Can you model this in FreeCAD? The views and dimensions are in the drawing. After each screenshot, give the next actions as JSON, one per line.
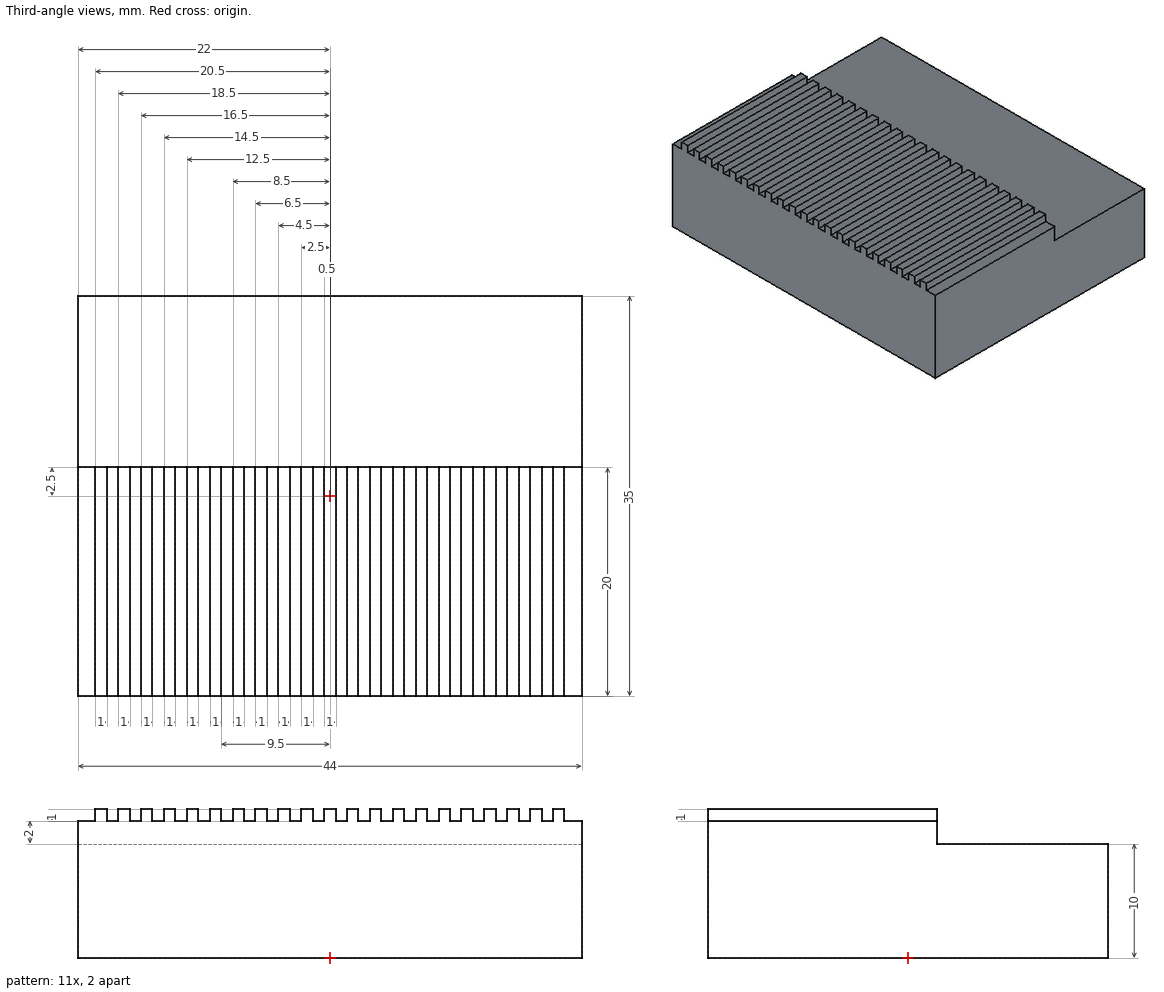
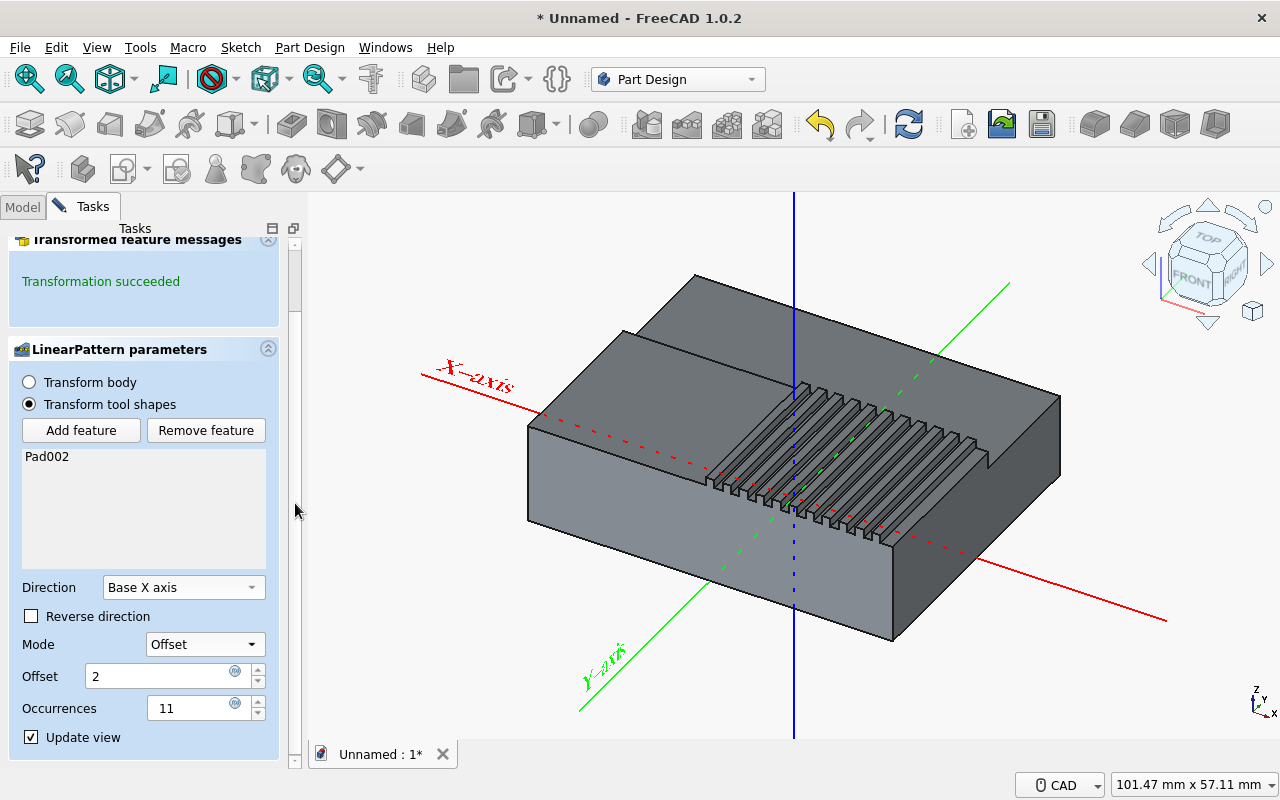
{"action": "left_click", "coordinate": [96, 267]}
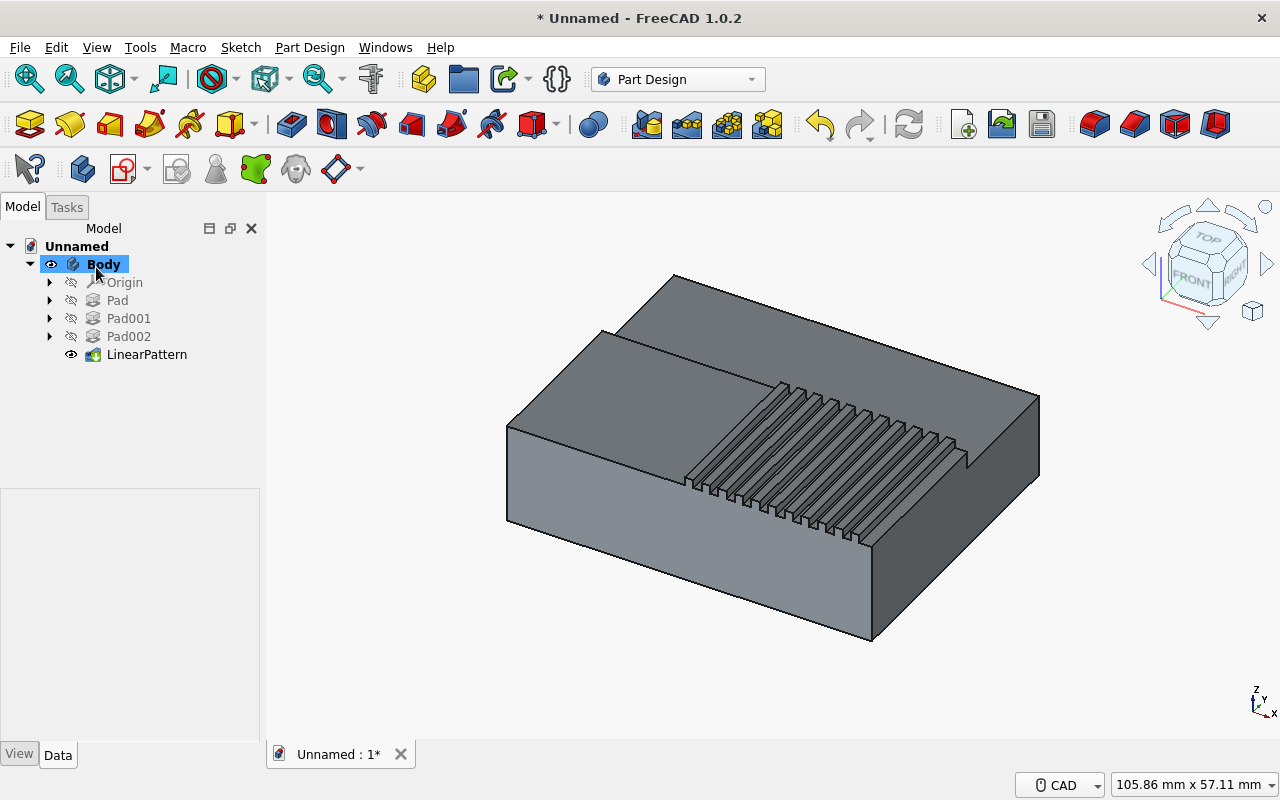
{"action": "left_click", "coordinate": [644, 407]}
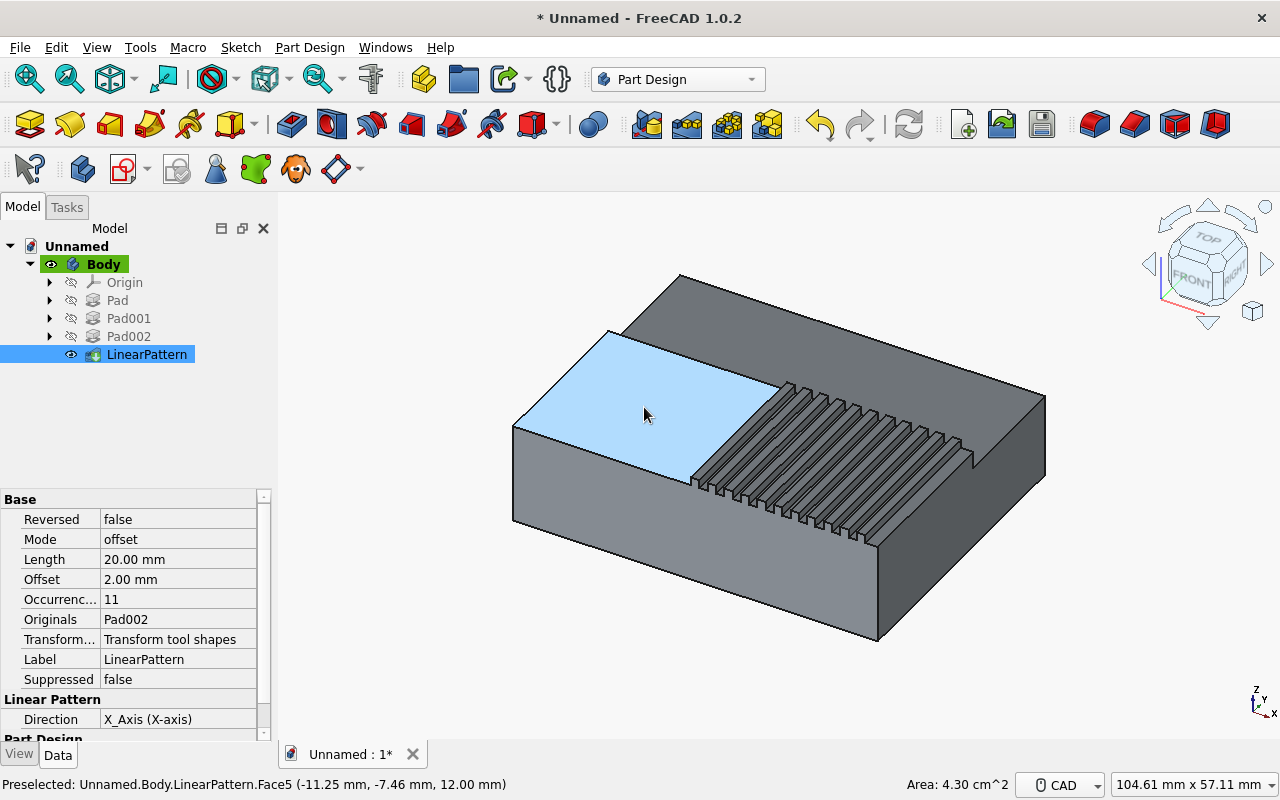
{"action": "left_click", "coordinate": [124, 170]}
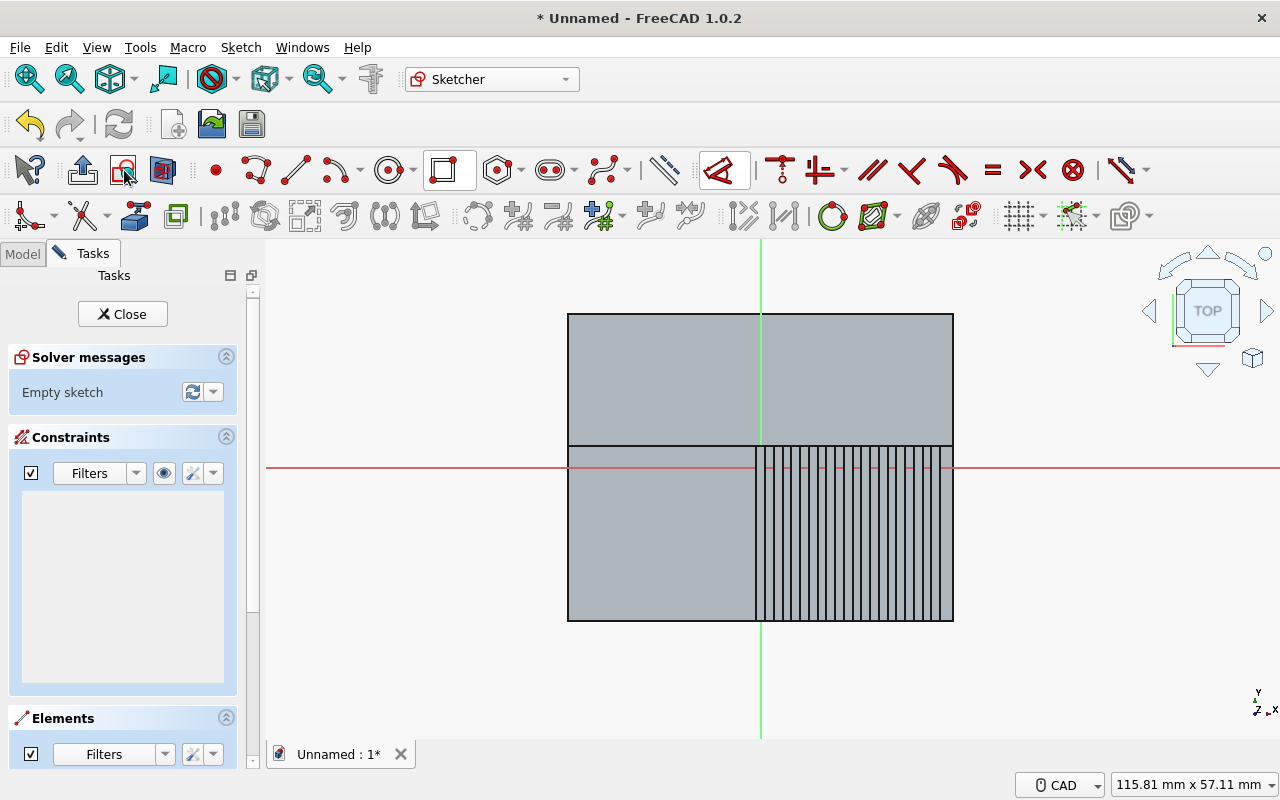
{"action": "left_click", "coordinate": [164, 170]}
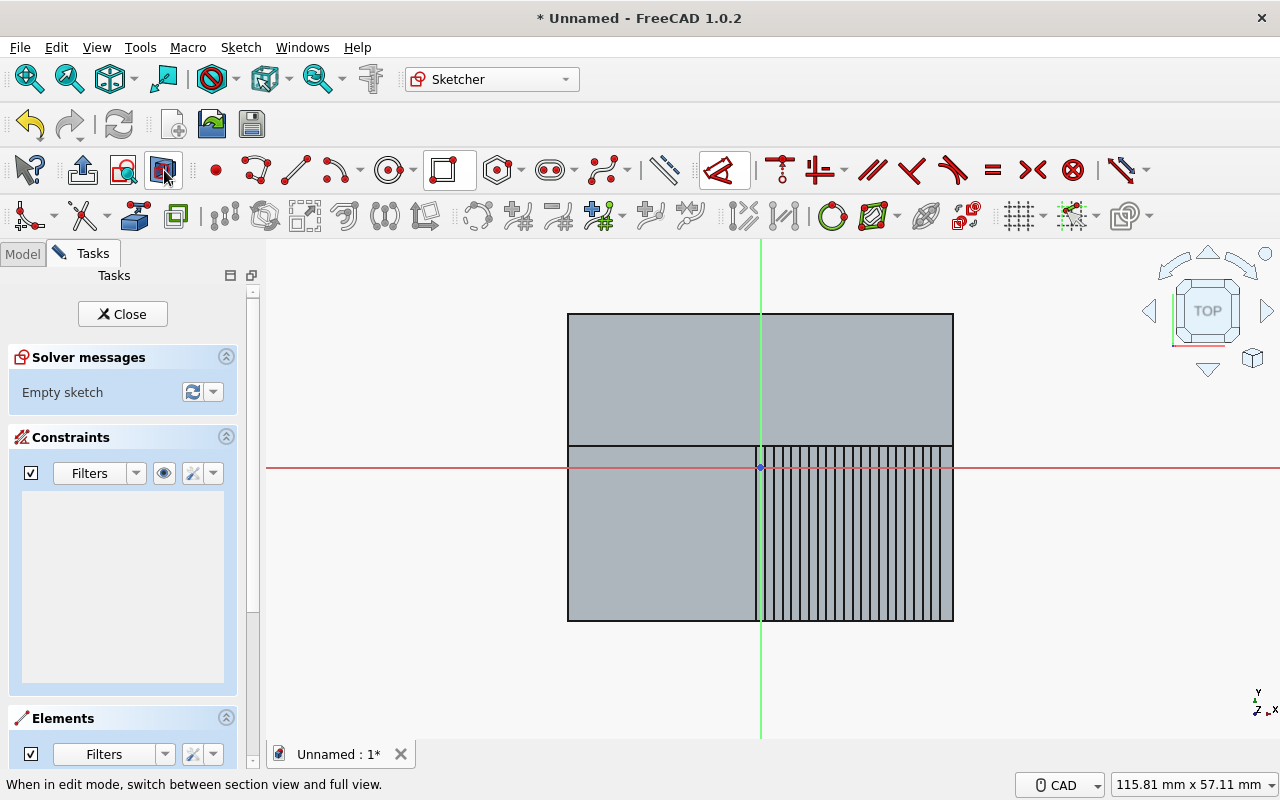
{"action": "scroll", "coordinate": [805, 587], "scroll_direction": "up", "scroll_amount": 3}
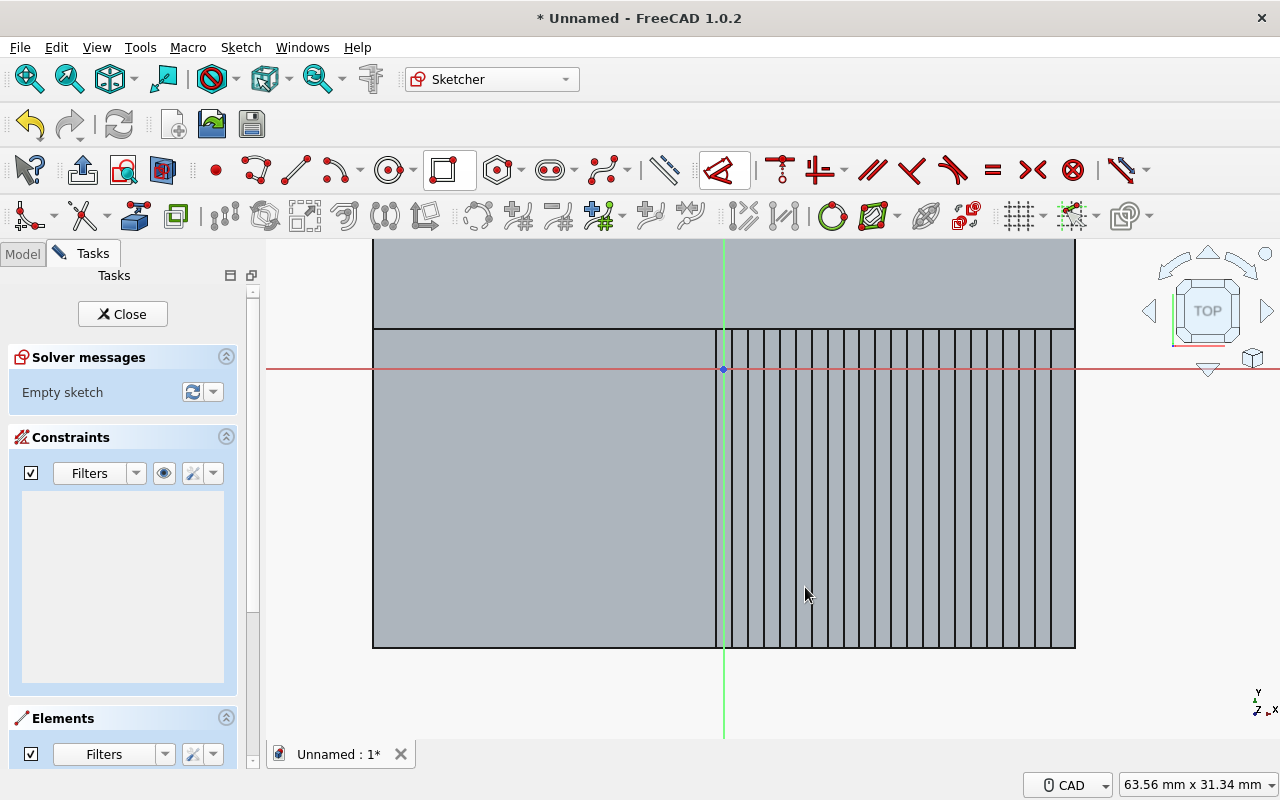
{"action": "left_click", "coordinate": [444, 170]}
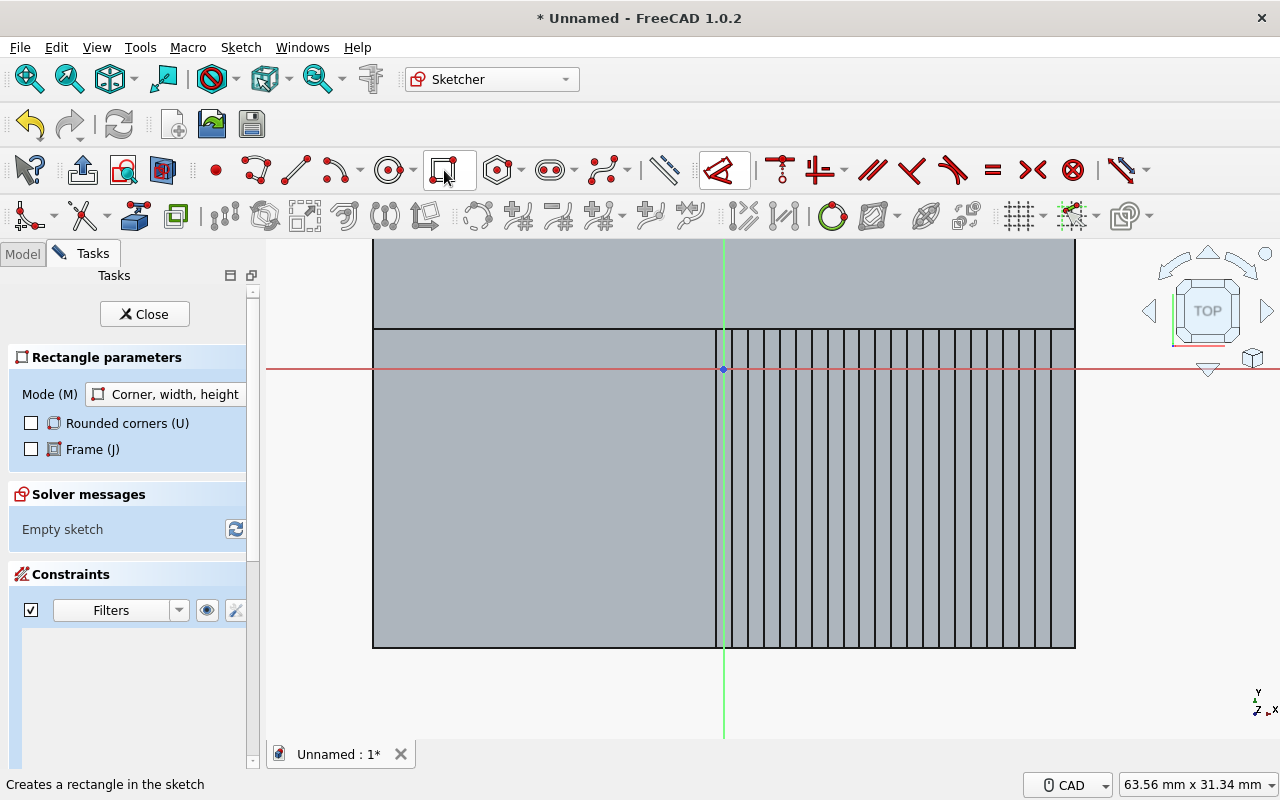
{"action": "left_click", "coordinate": [684, 329]}
{"action": "mouse_move", "coordinate": [700, 648]}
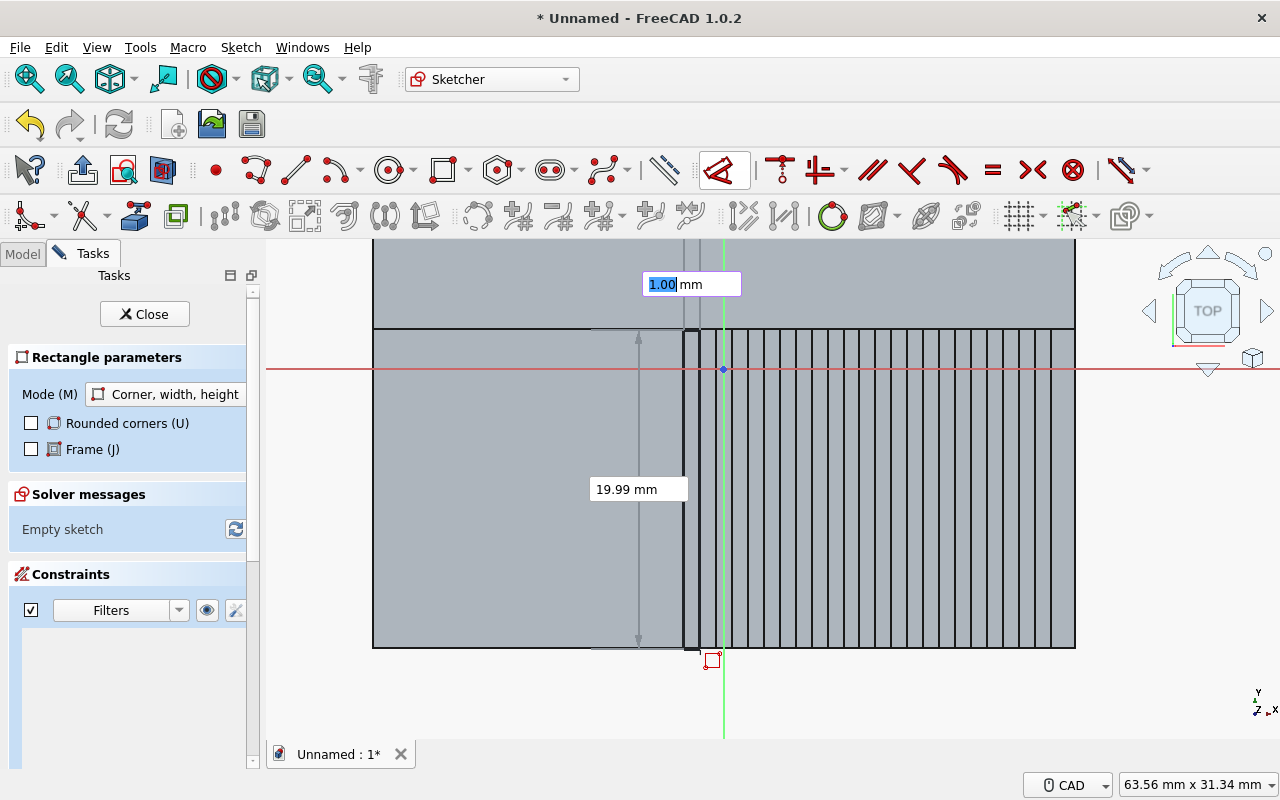
{"action": "type", "text": "1"}
{"action": "key", "text": "Tab"}
{"action": "type", "text": "20"}
{"action": "key", "text": "Return"}
{"action": "key", "text": "Escape"}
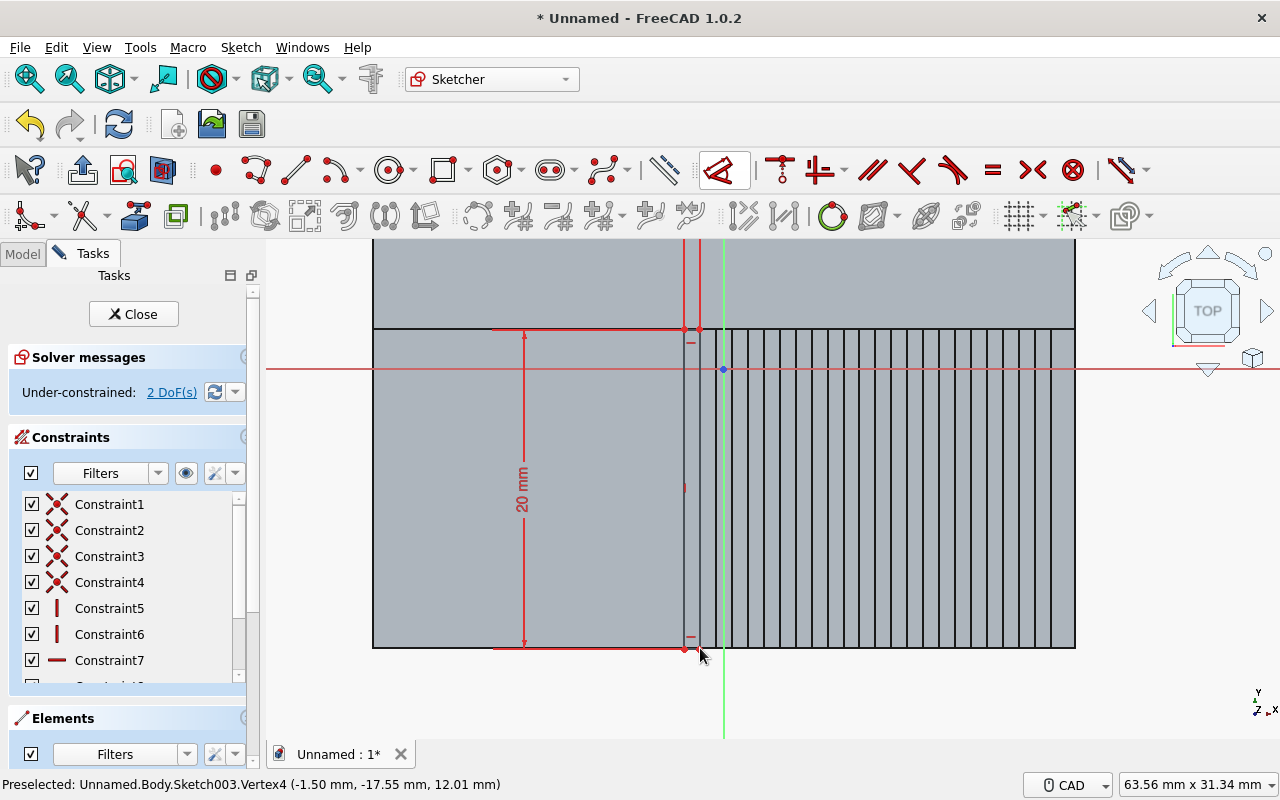
{"action": "left_click", "coordinate": [684, 330]}